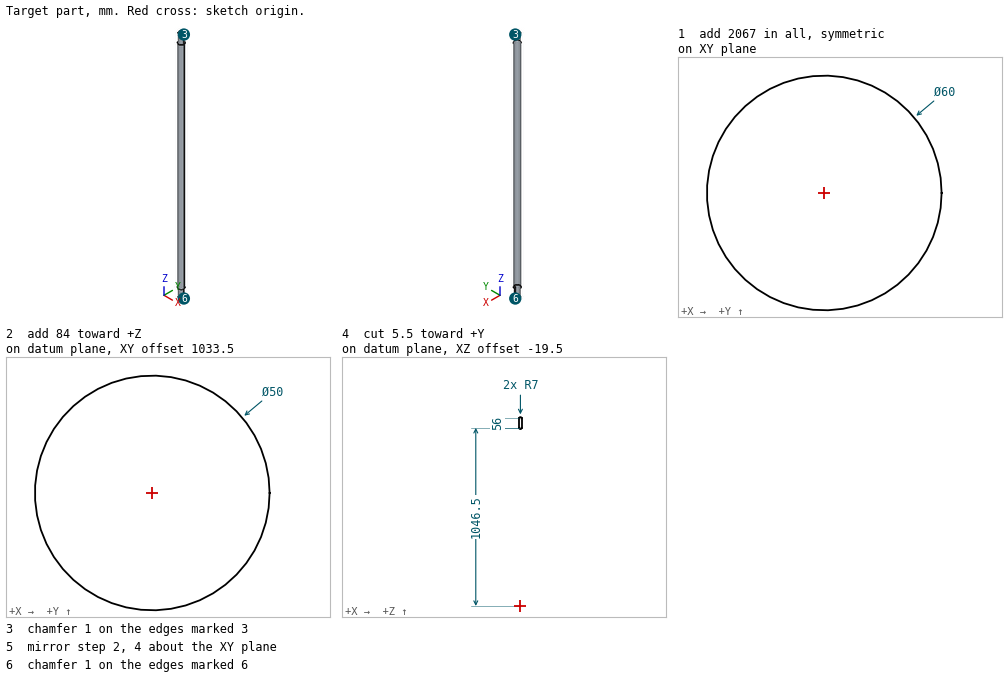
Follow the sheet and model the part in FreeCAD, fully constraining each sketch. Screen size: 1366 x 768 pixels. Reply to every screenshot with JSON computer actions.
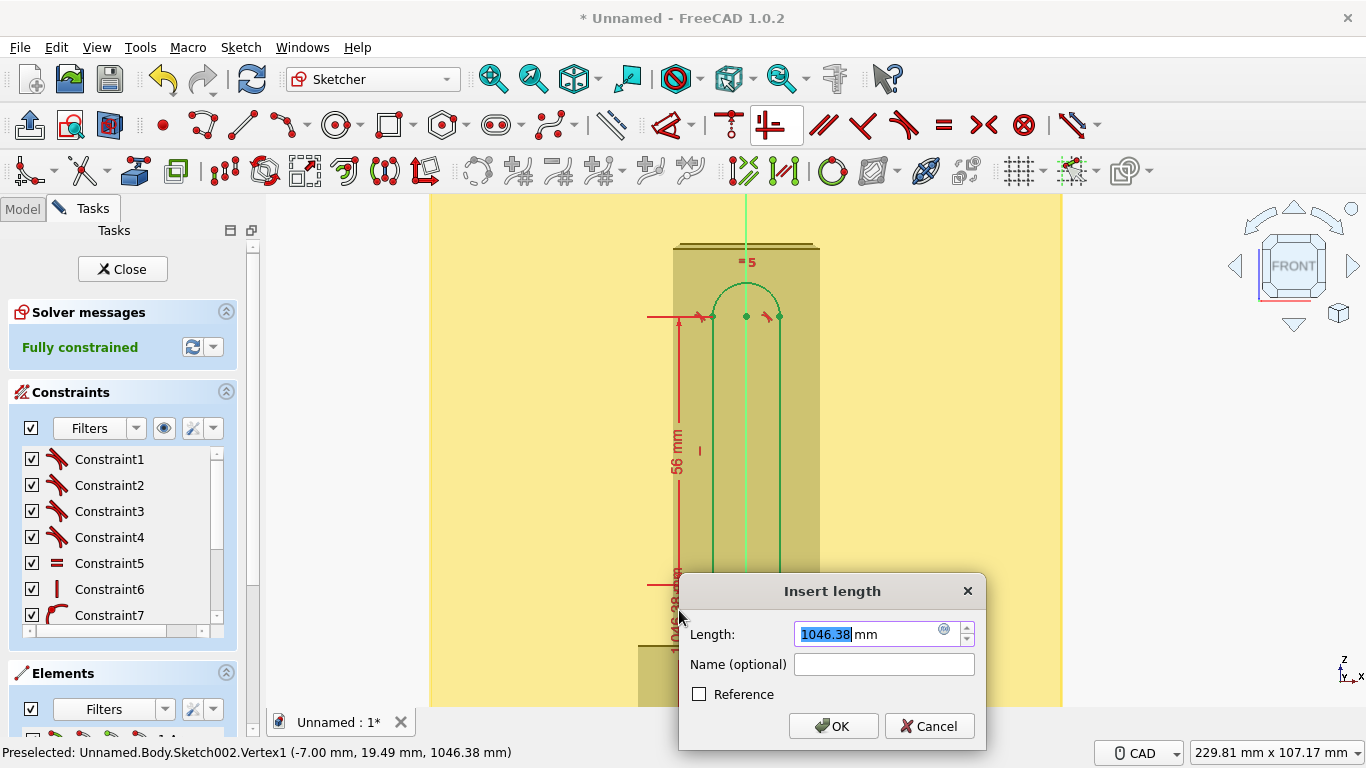
{"action": "type", "text": "1046.5"}
{"action": "key", "text": "Return"}
{"action": "key", "text": "Escape"}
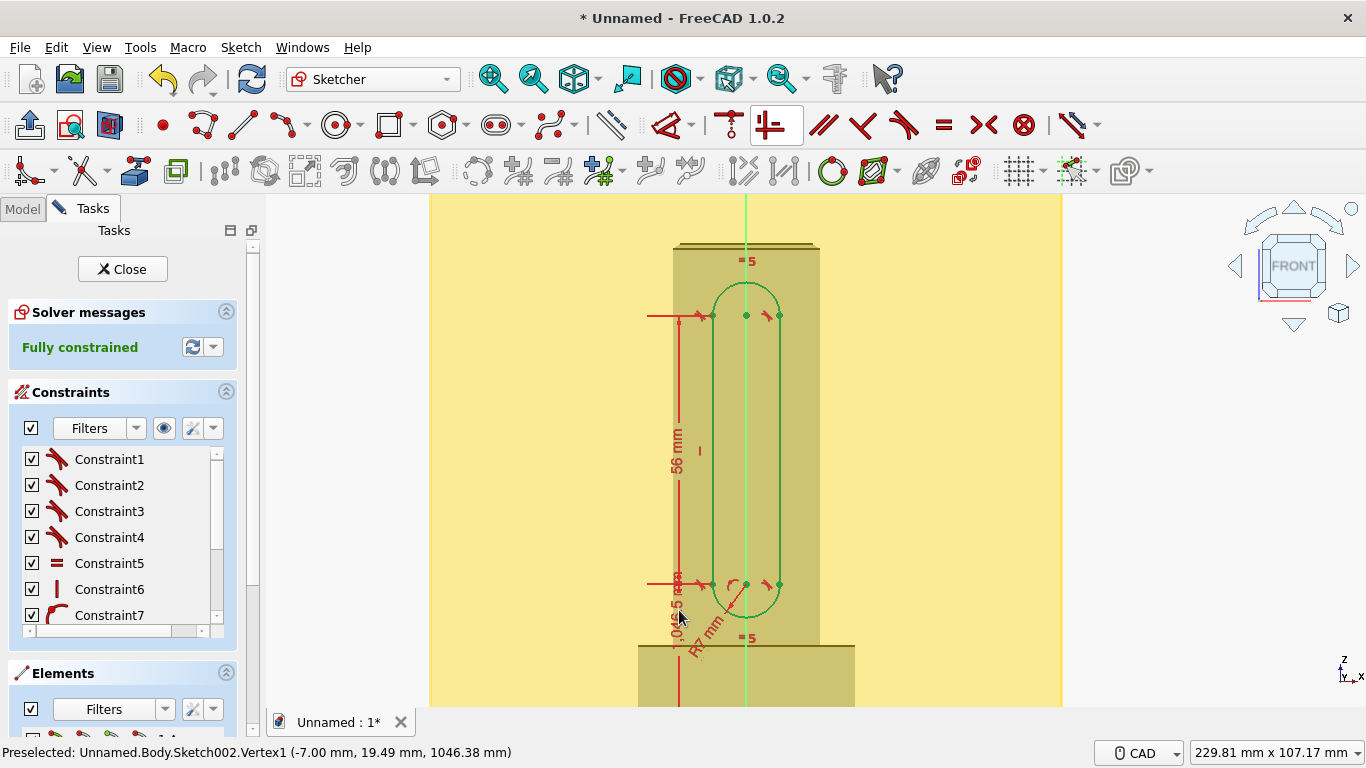
{"action": "left_click", "coordinate": [123, 269]}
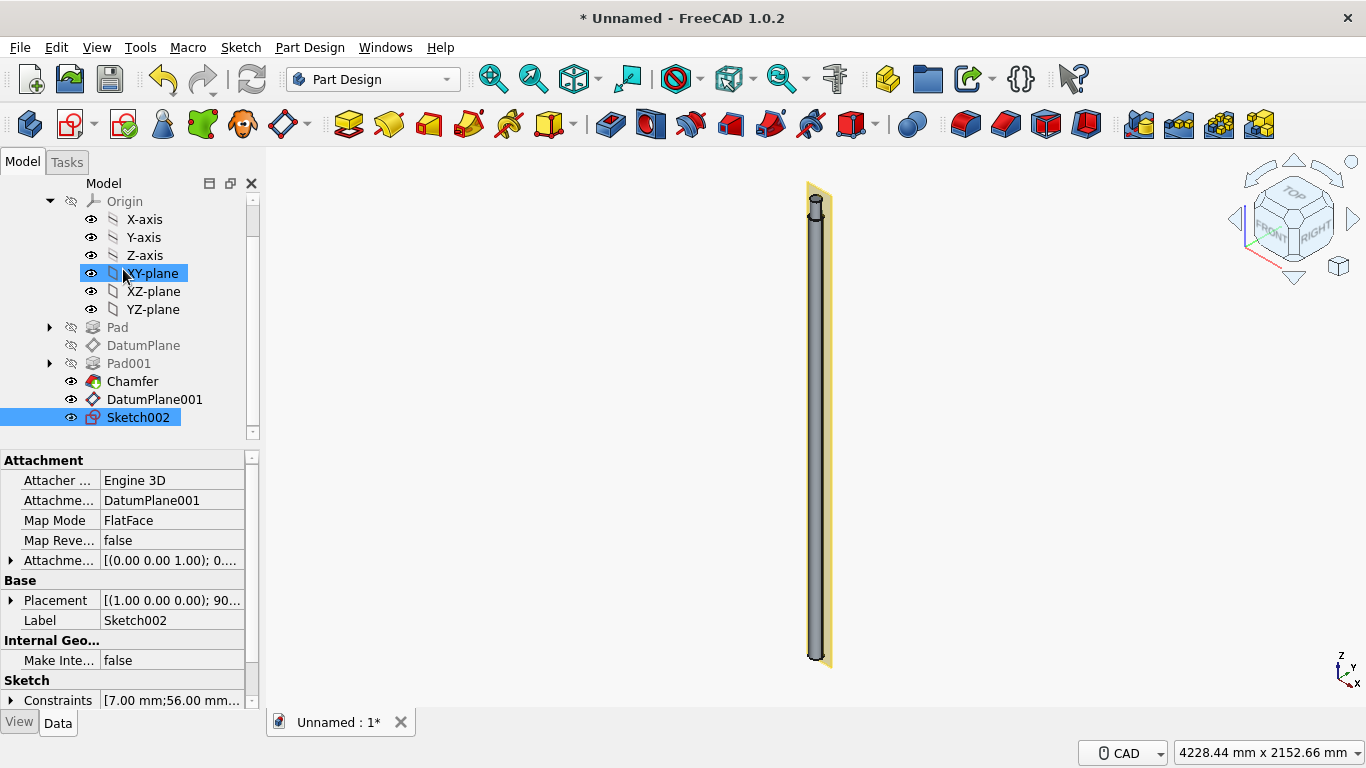
{"action": "left_click", "coordinate": [612, 124]}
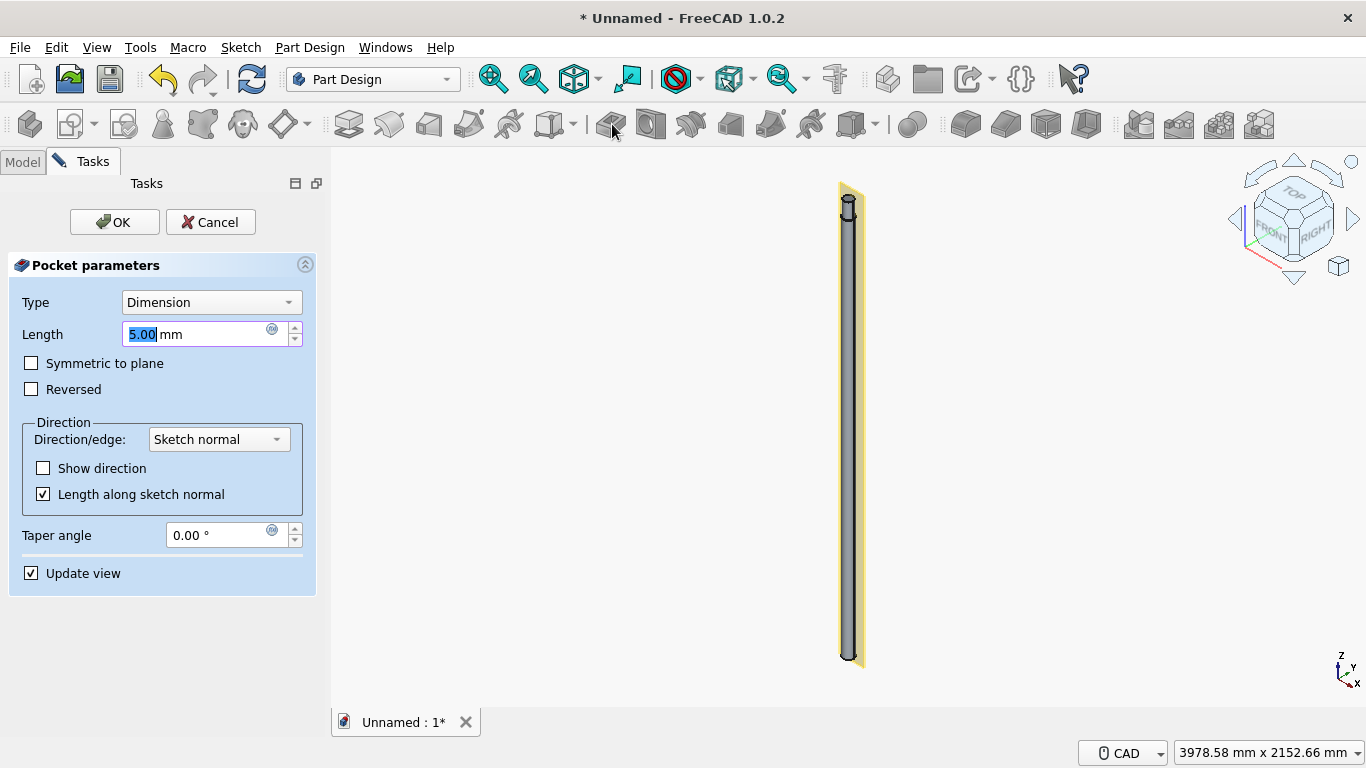
{"action": "type", "text": "5.5"}
{"action": "key", "text": "Tab"}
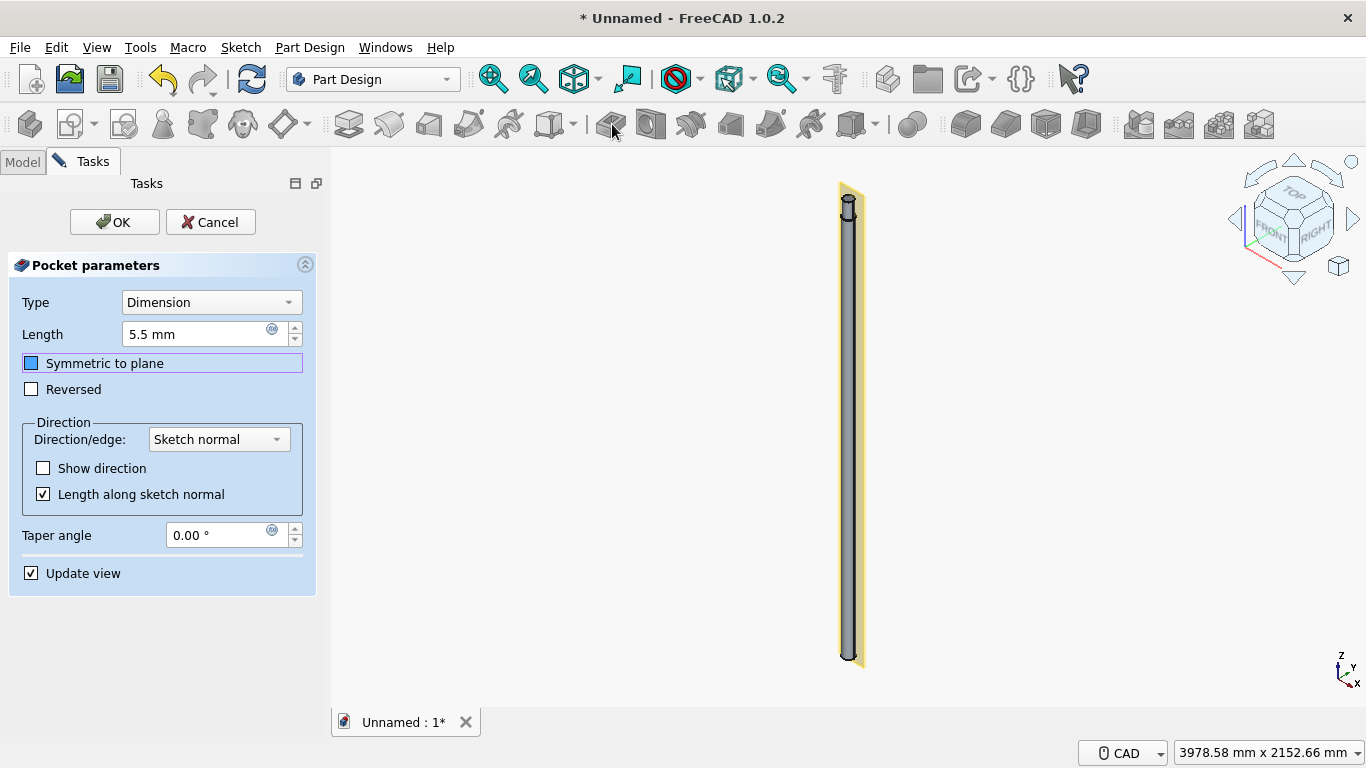
{"action": "left_click", "coordinate": [115, 222]}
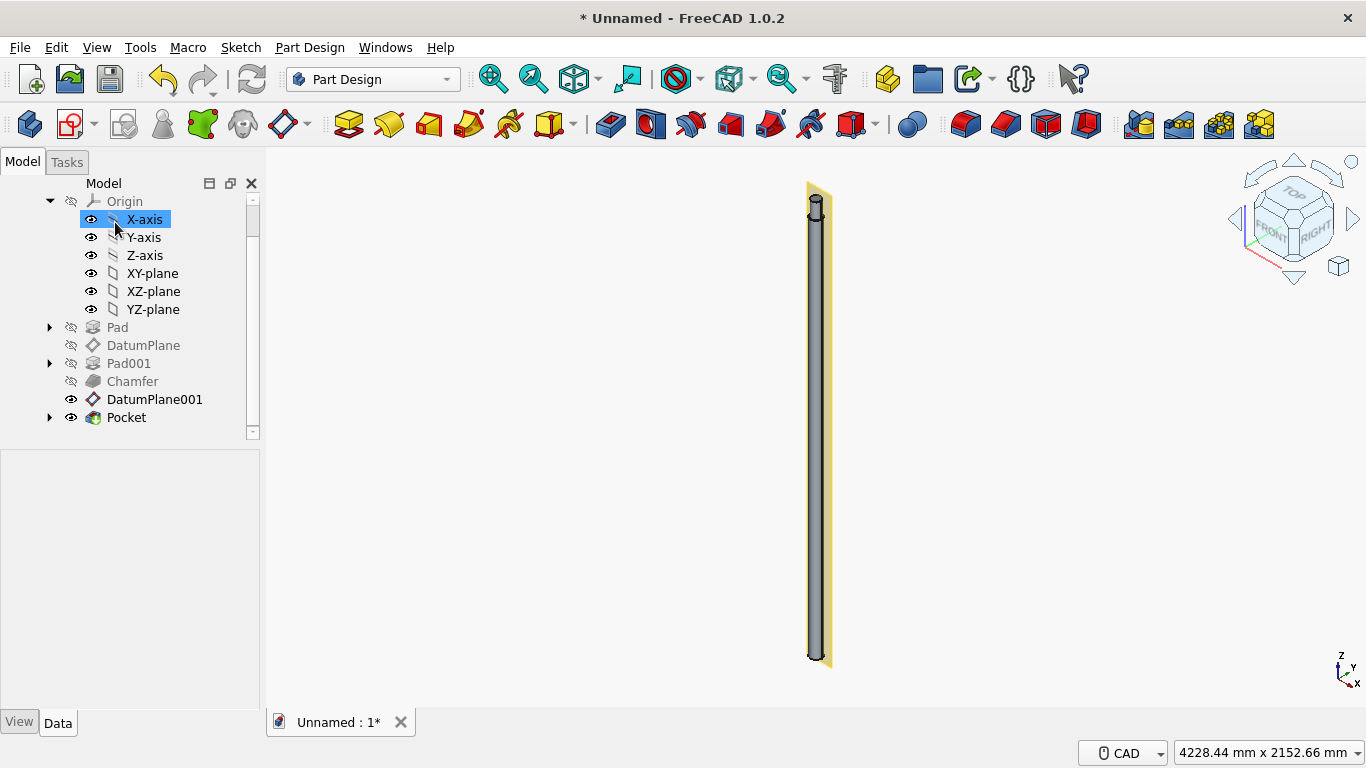
{"action": "left_click", "coordinate": [116, 399]}
{"action": "key", "text": "space"}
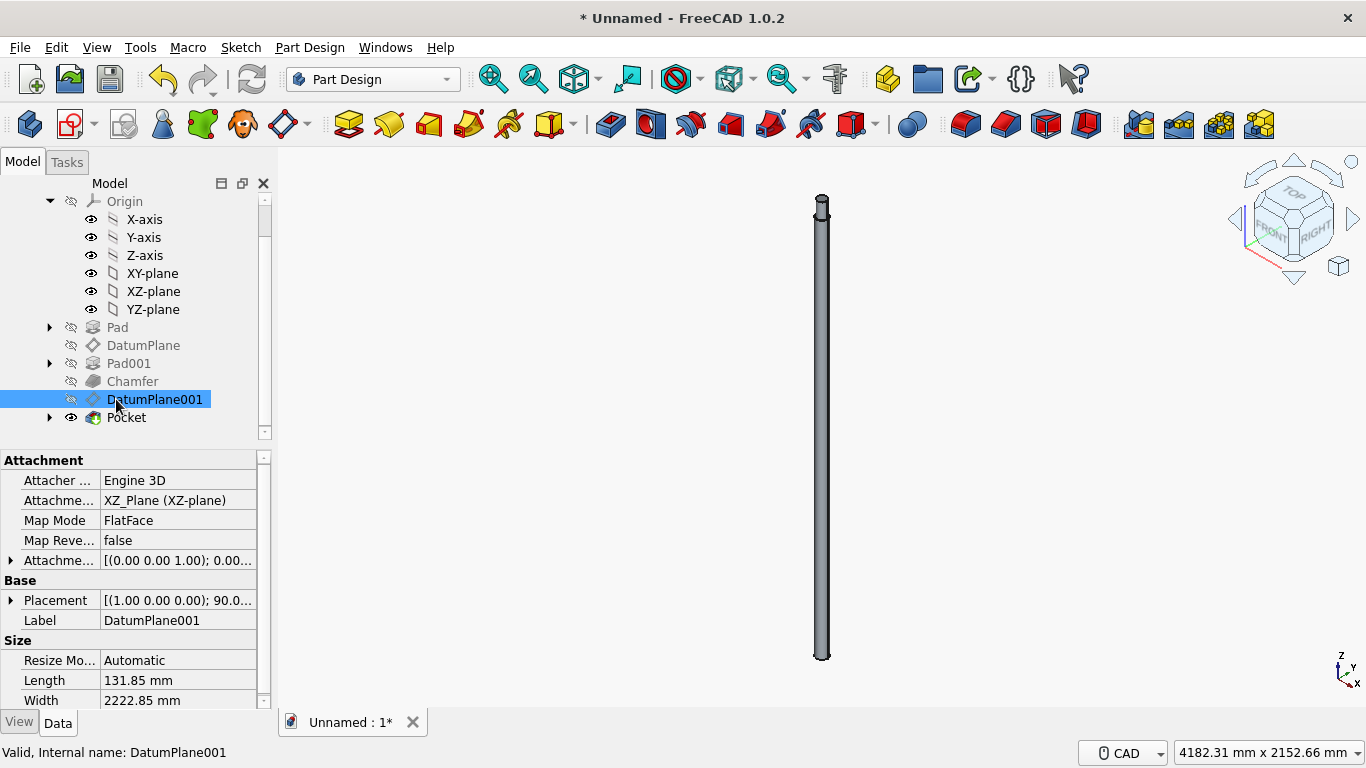
{"action": "left_click", "coordinate": [116, 363]}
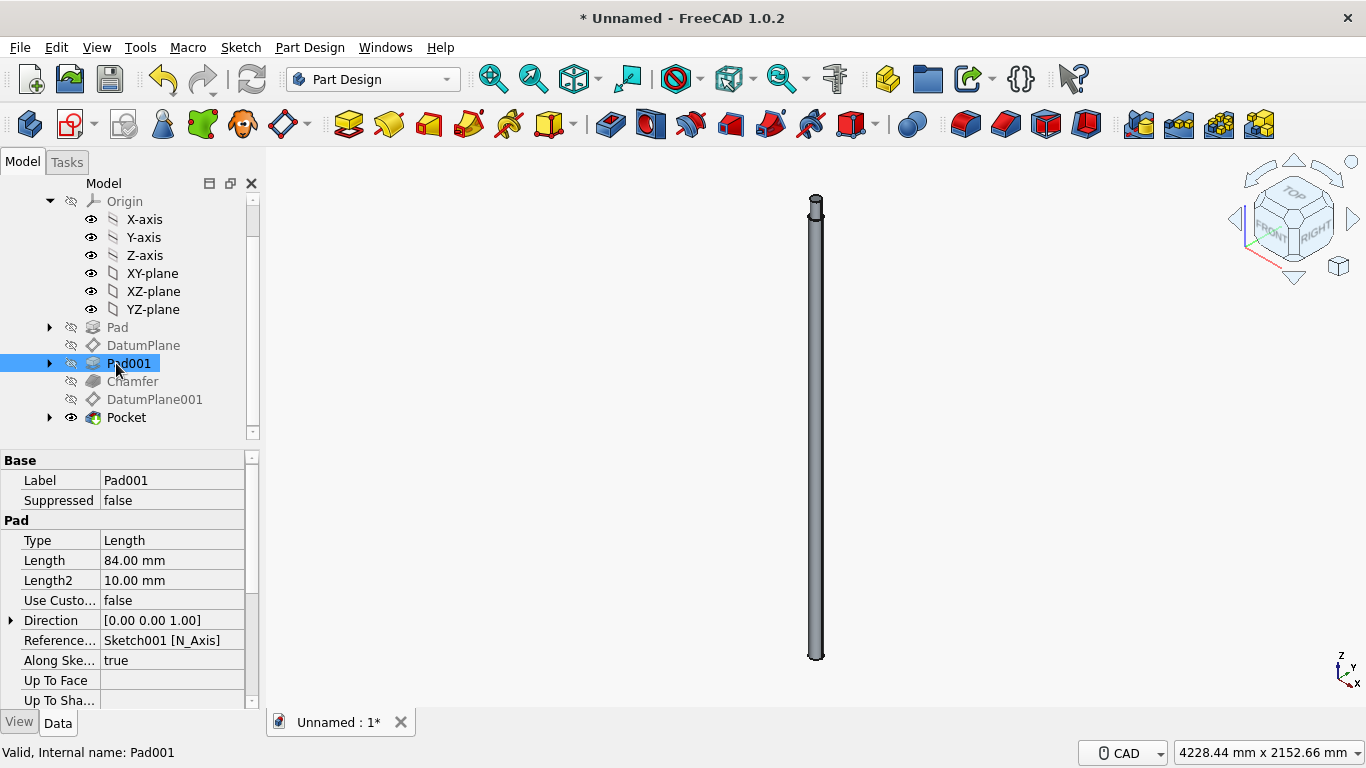
{"action": "left_click", "coordinate": [116, 417], "text": "ctrl"}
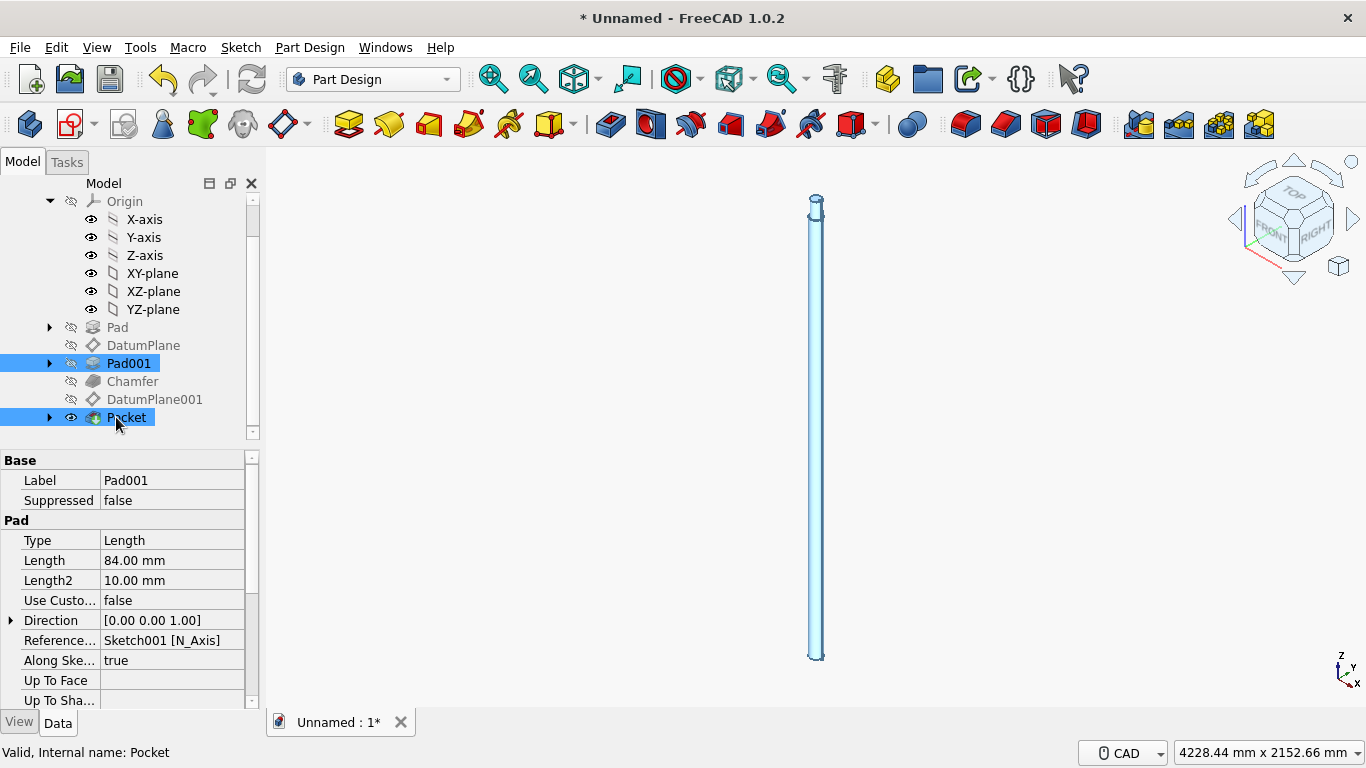
{"action": "left_click", "coordinate": [1140, 124]}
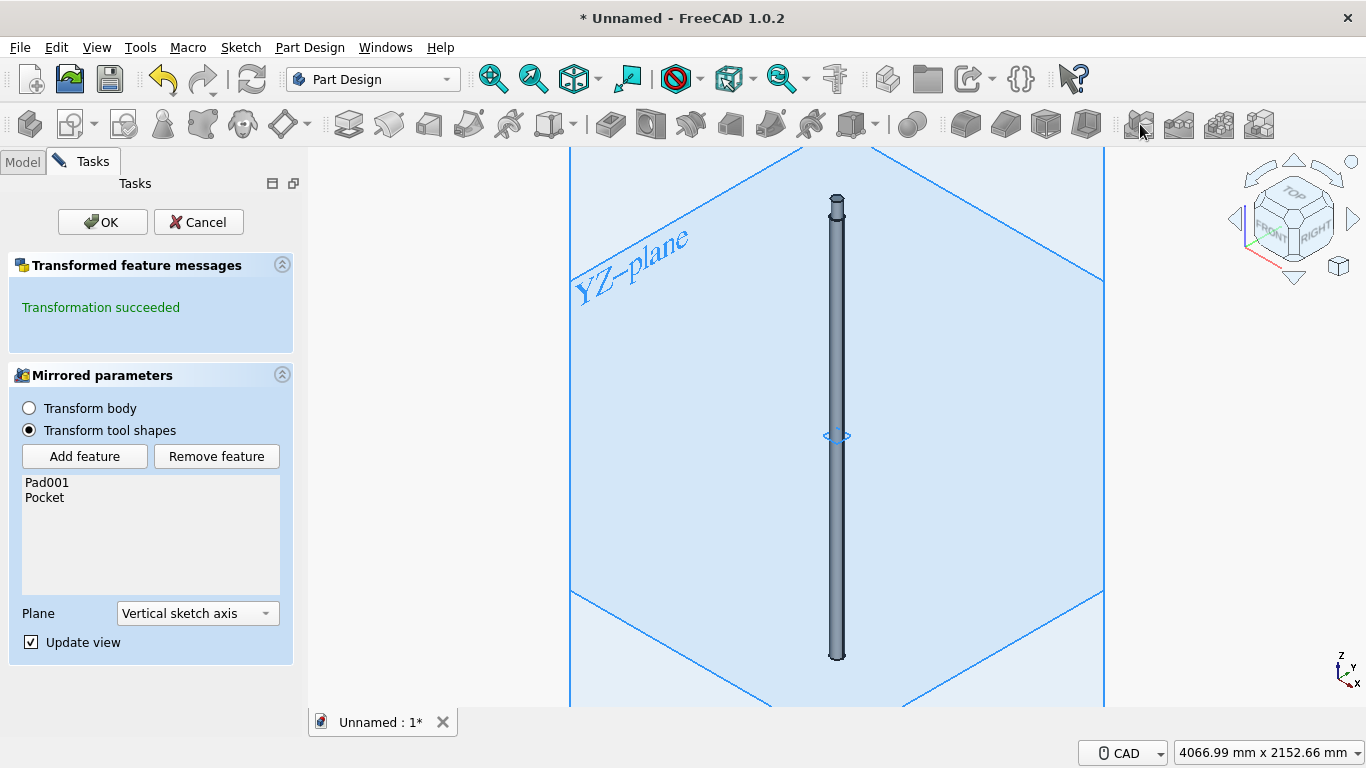
{"action": "left_click", "coordinate": [198, 614]}